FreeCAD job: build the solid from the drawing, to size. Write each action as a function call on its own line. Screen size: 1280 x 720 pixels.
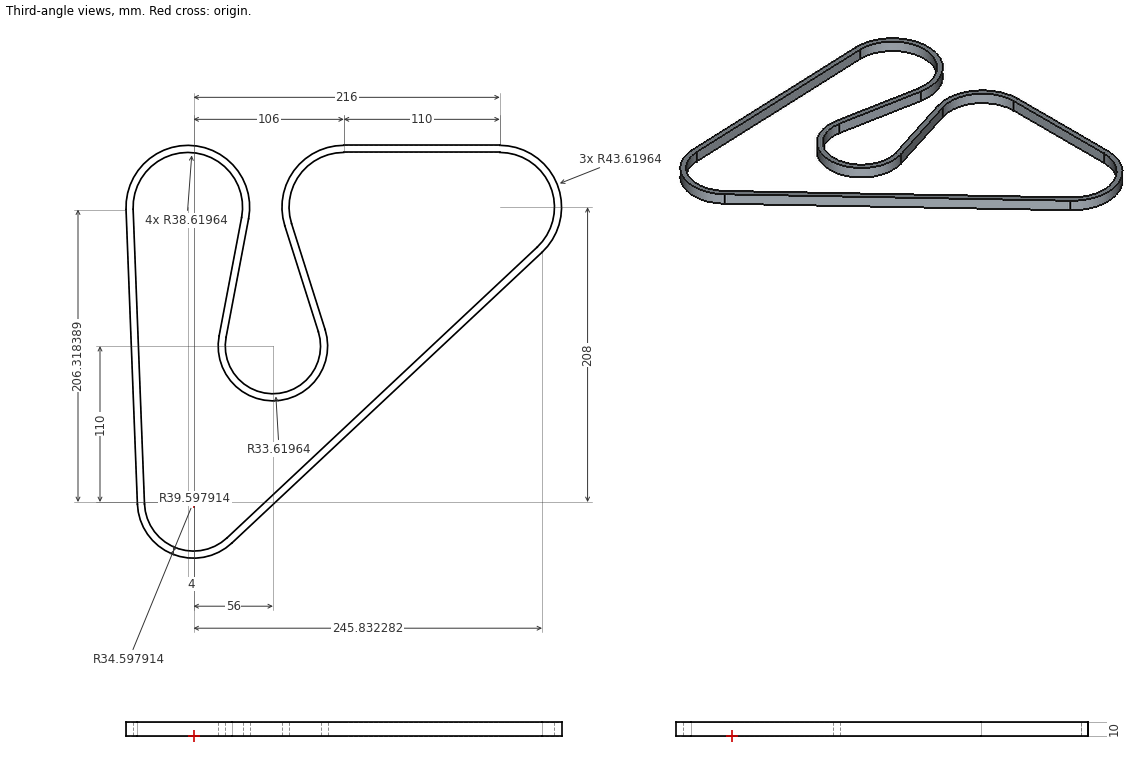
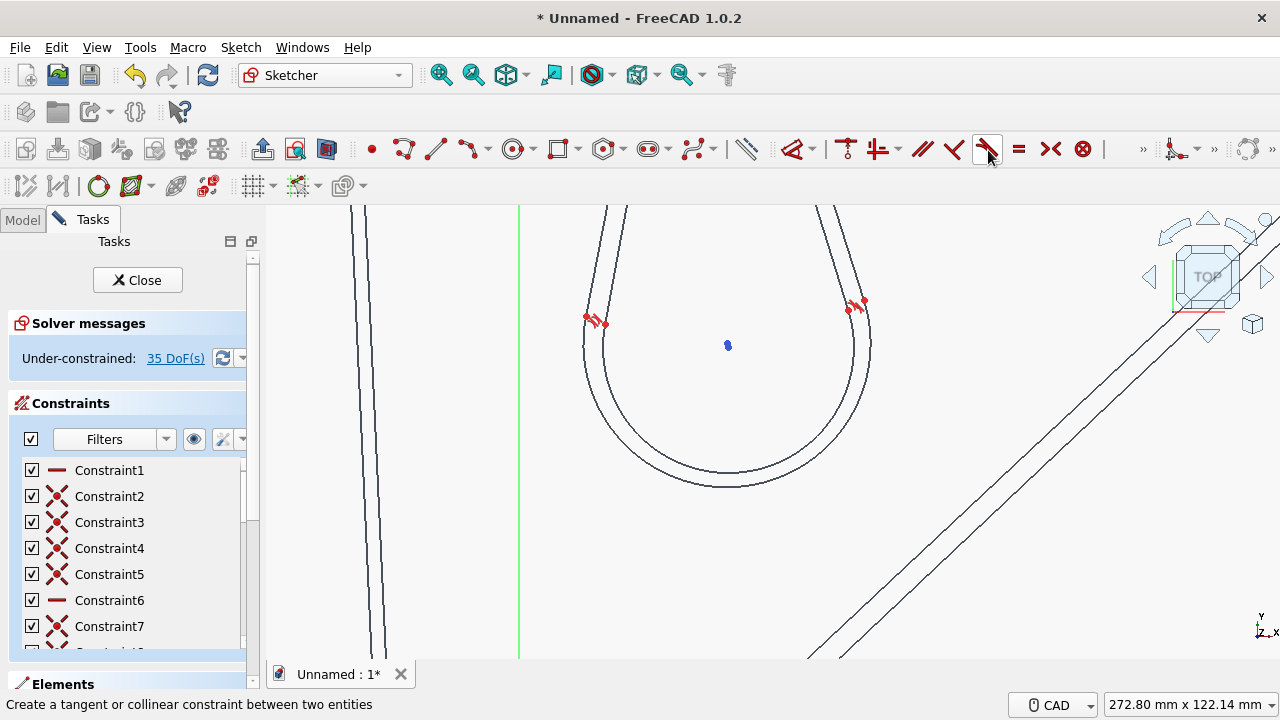
click(847, 245)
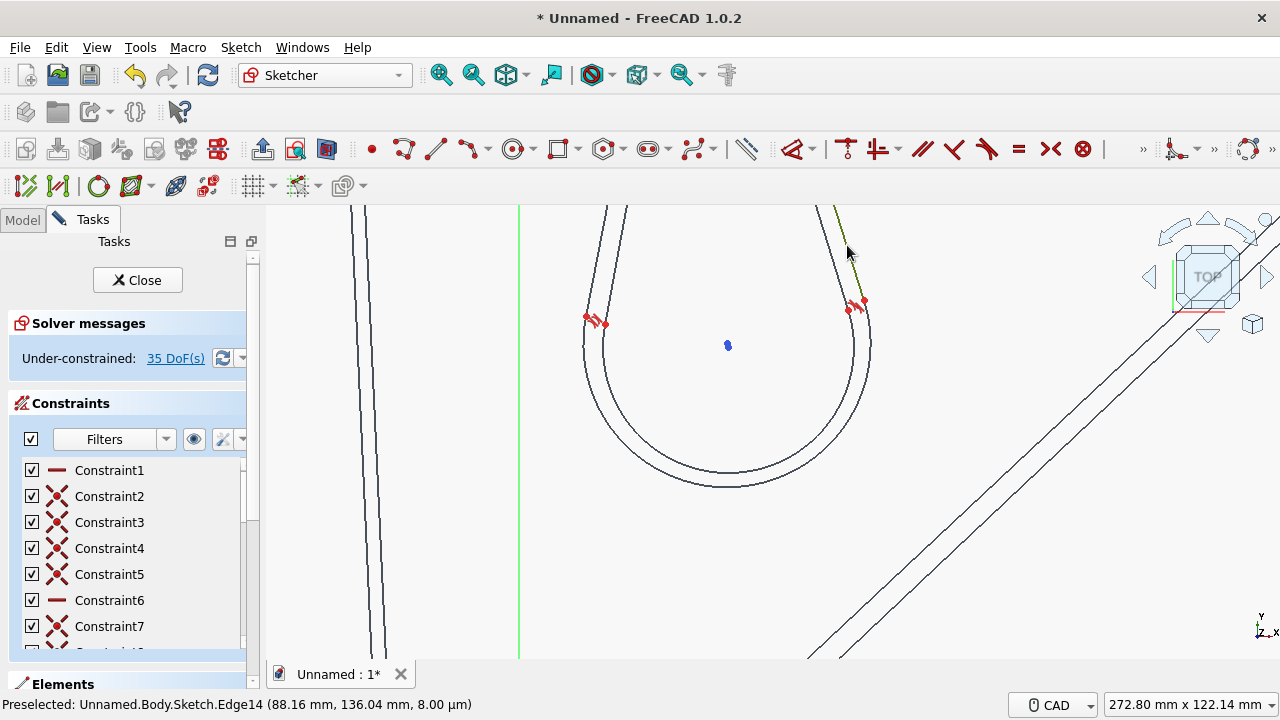
scroll(638, 458, down, 7)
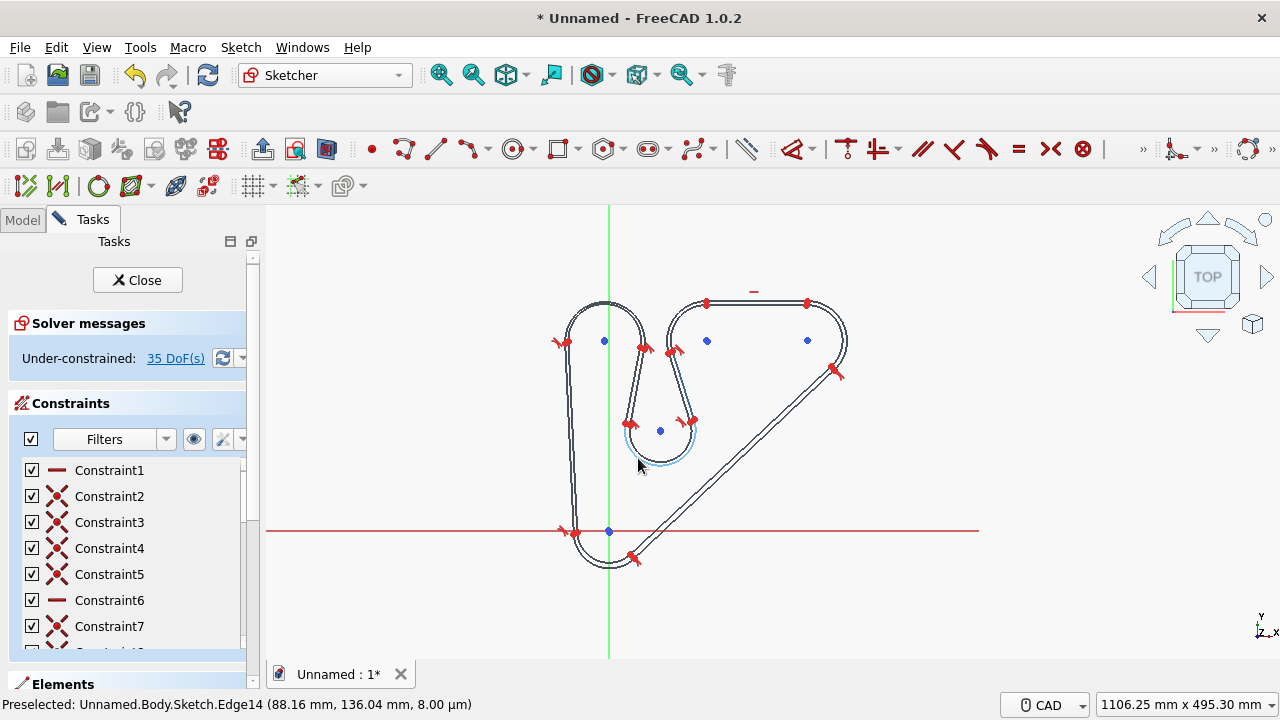
scroll(687, 311, up, 7)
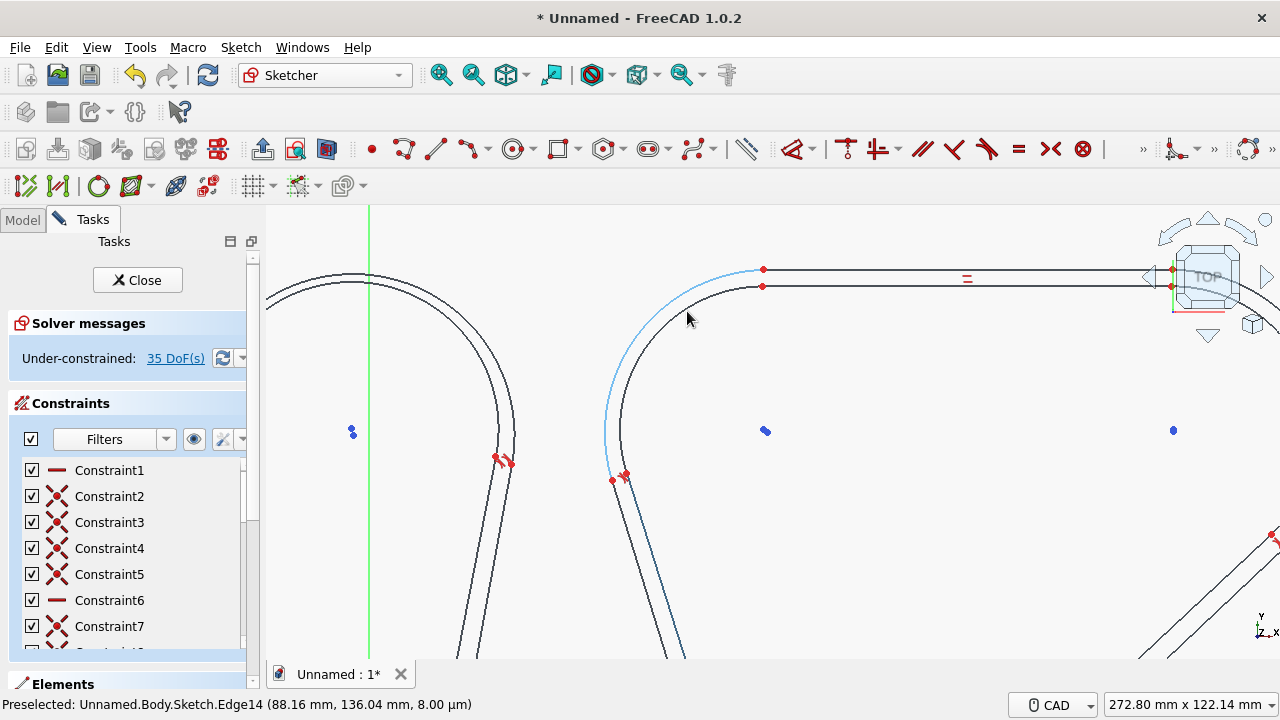
click(686, 309)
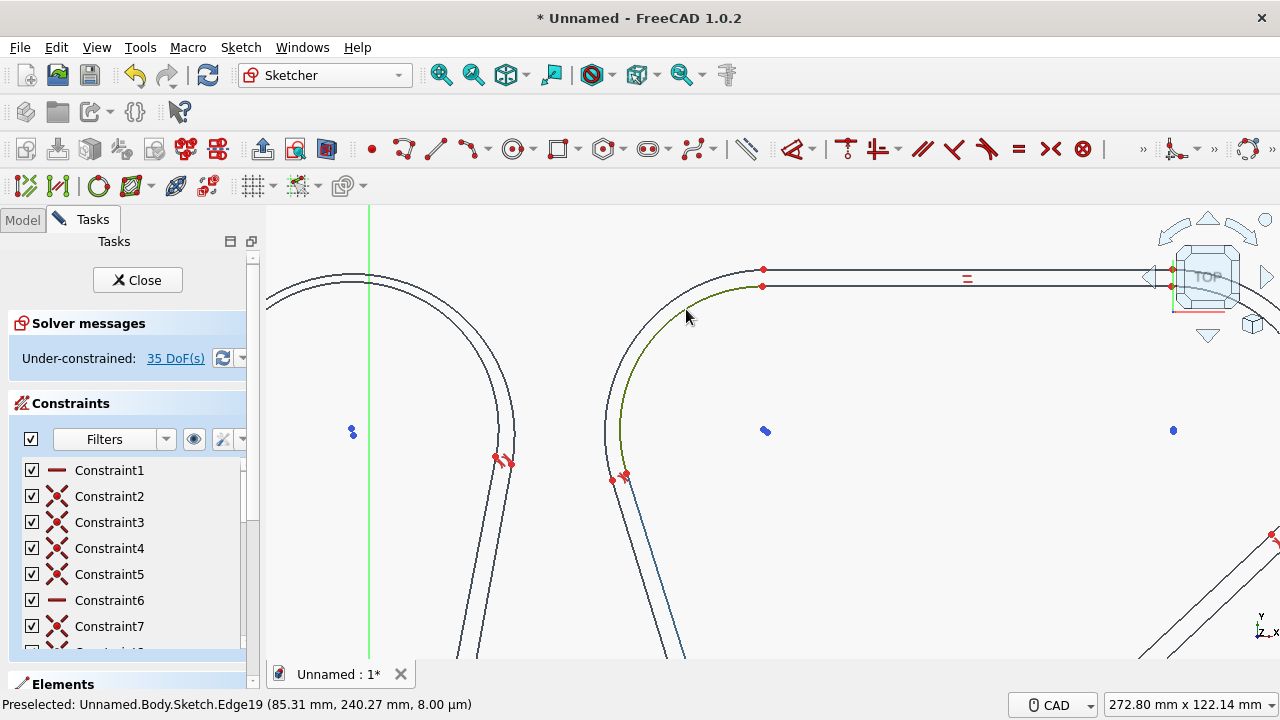
click(988, 150)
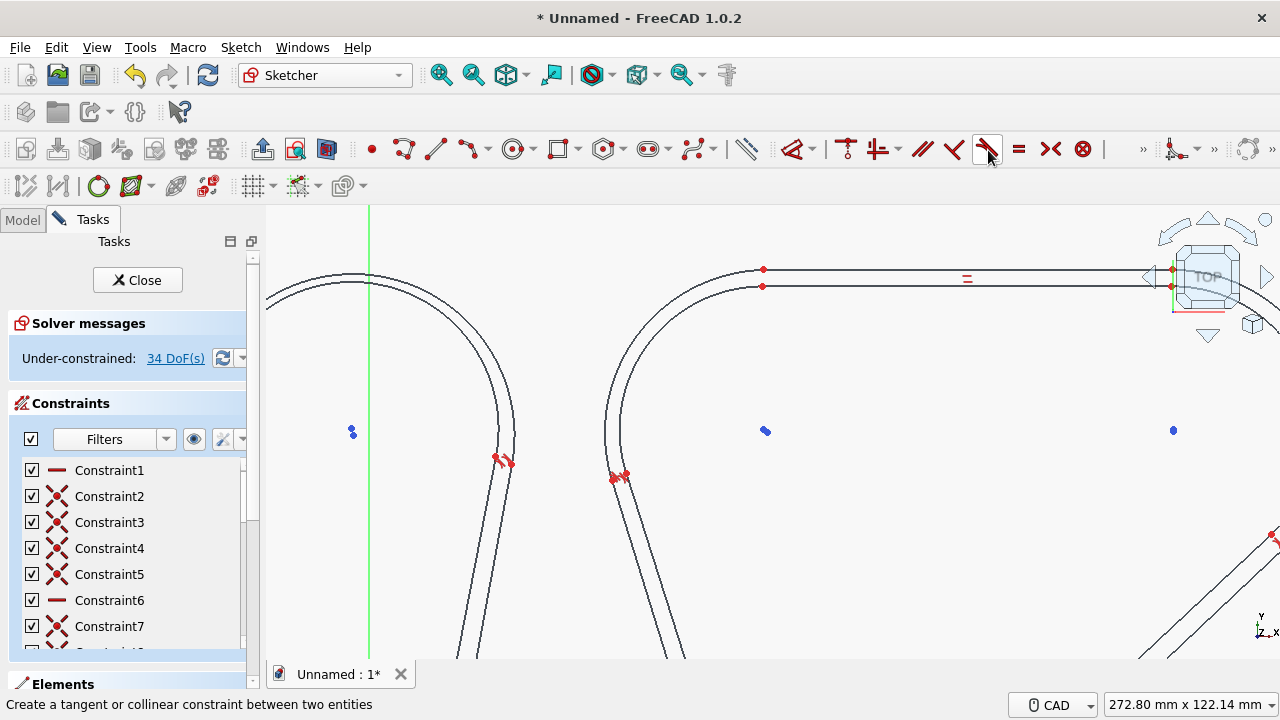
click(886, 286)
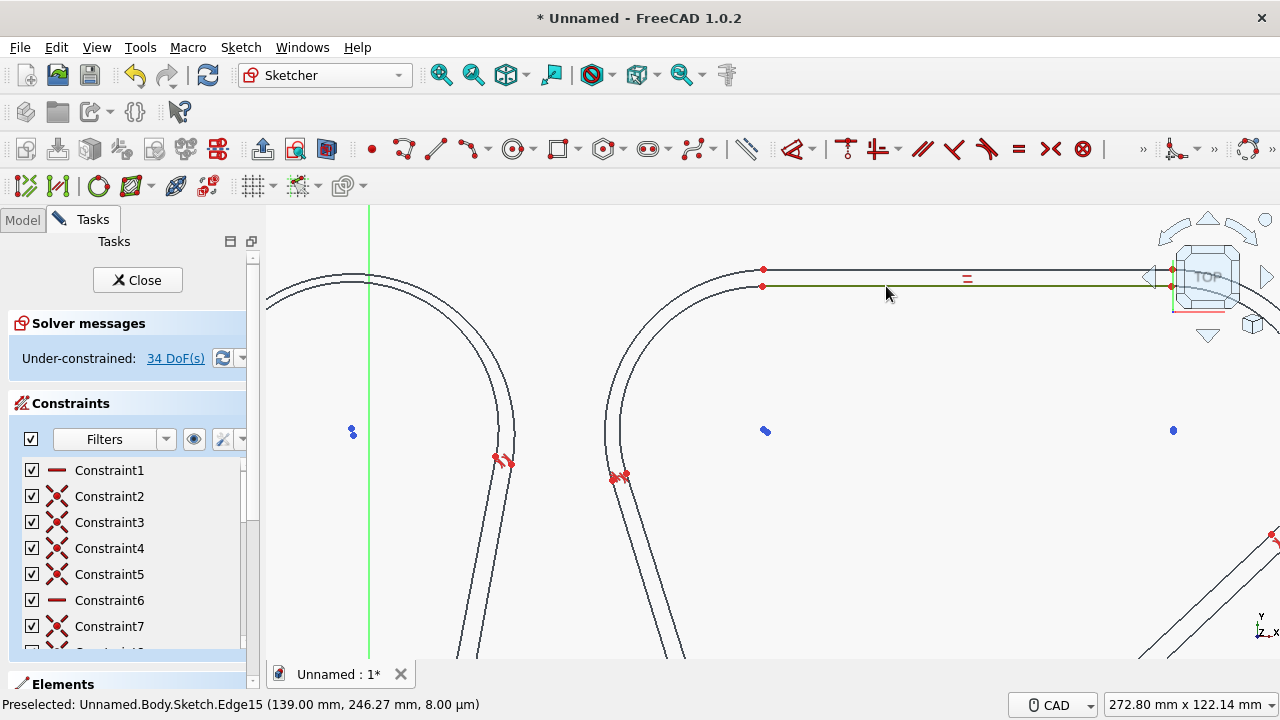
click(686, 309)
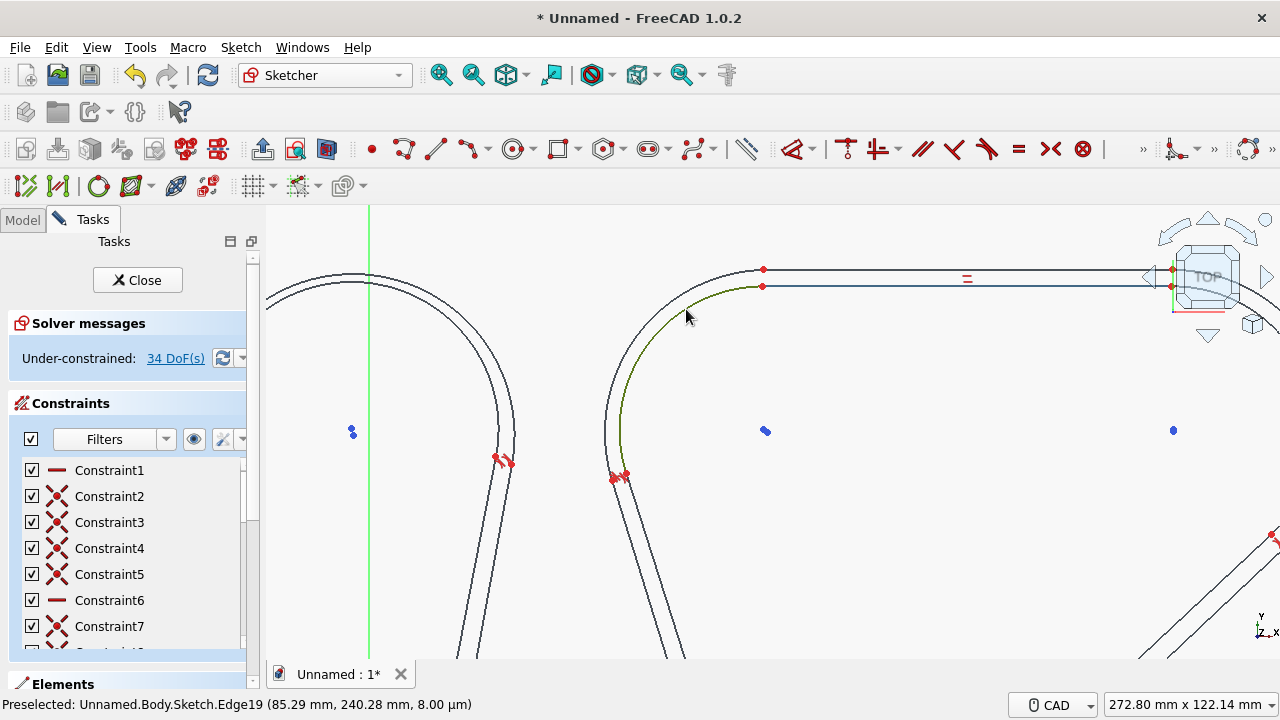
click(988, 150)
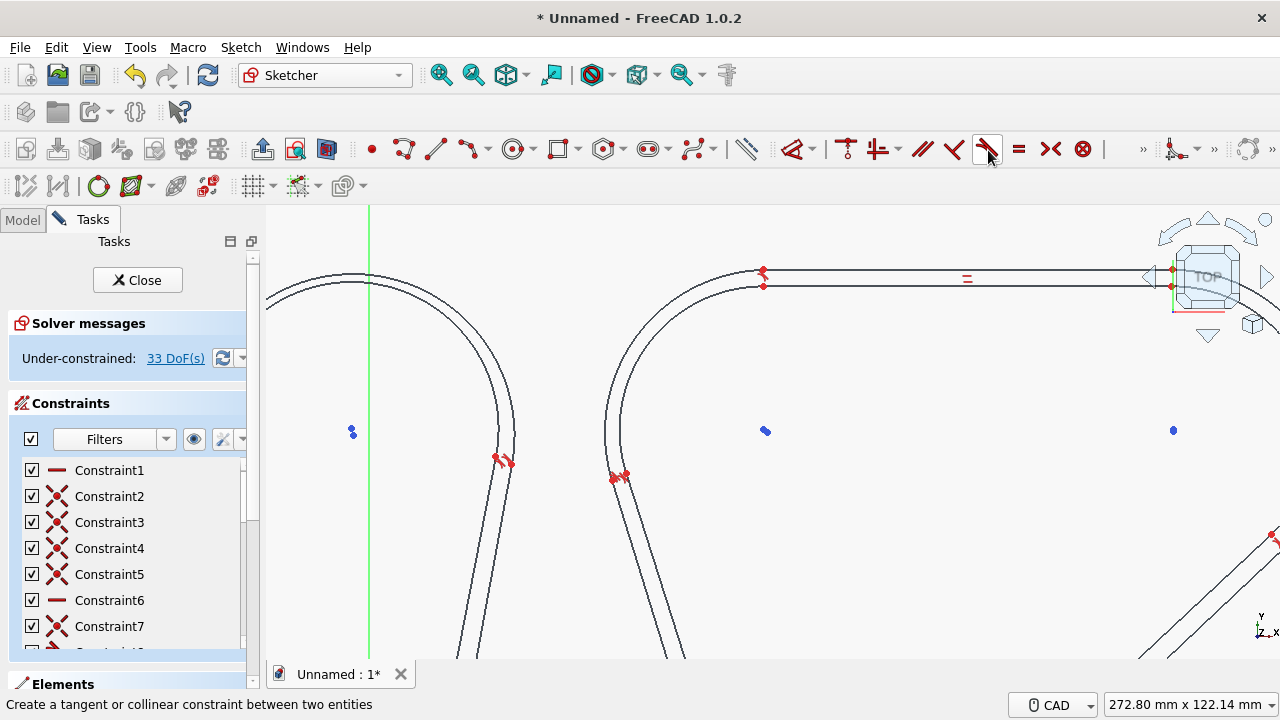
click(886, 286)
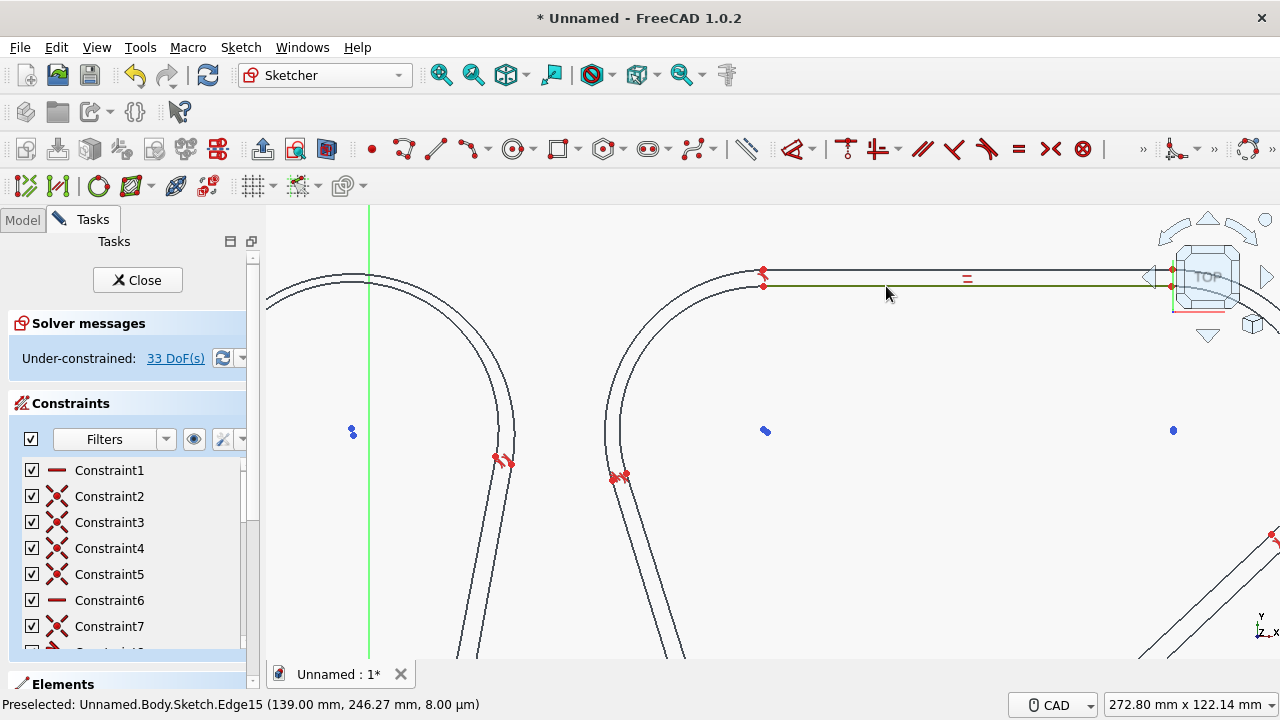
scroll(687, 311, down, 7)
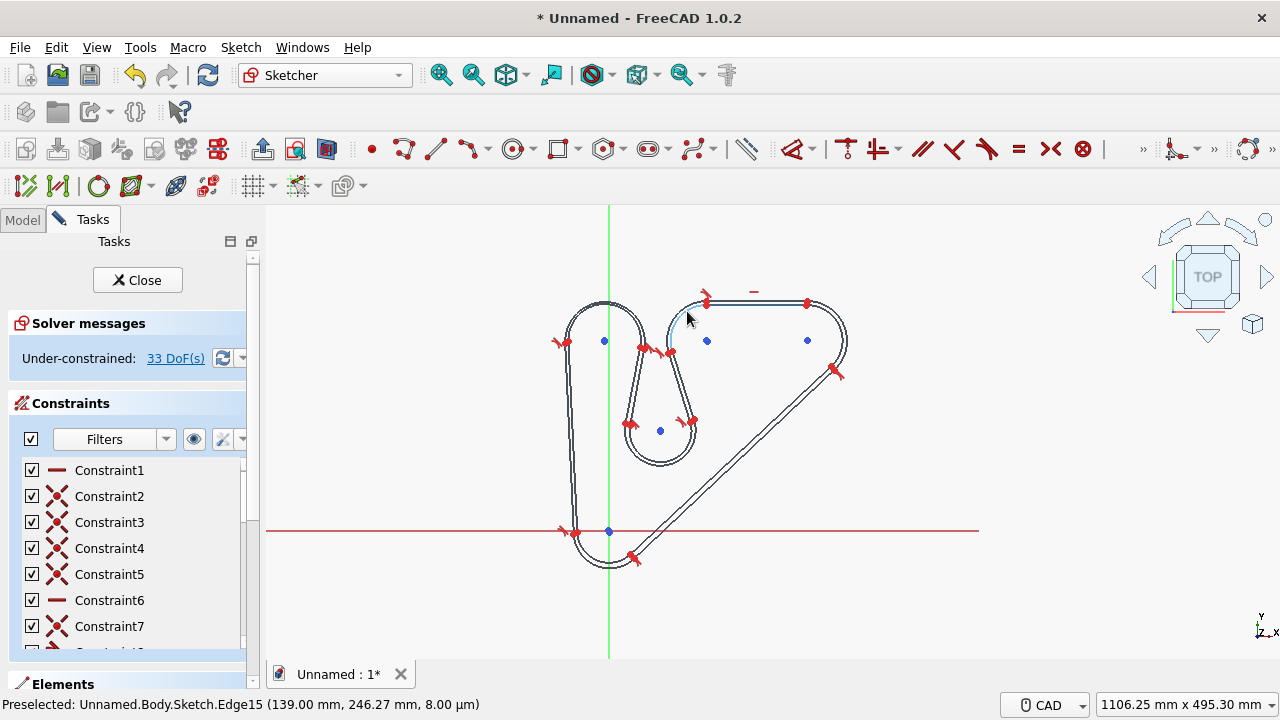
scroll(842, 344, up, 6)